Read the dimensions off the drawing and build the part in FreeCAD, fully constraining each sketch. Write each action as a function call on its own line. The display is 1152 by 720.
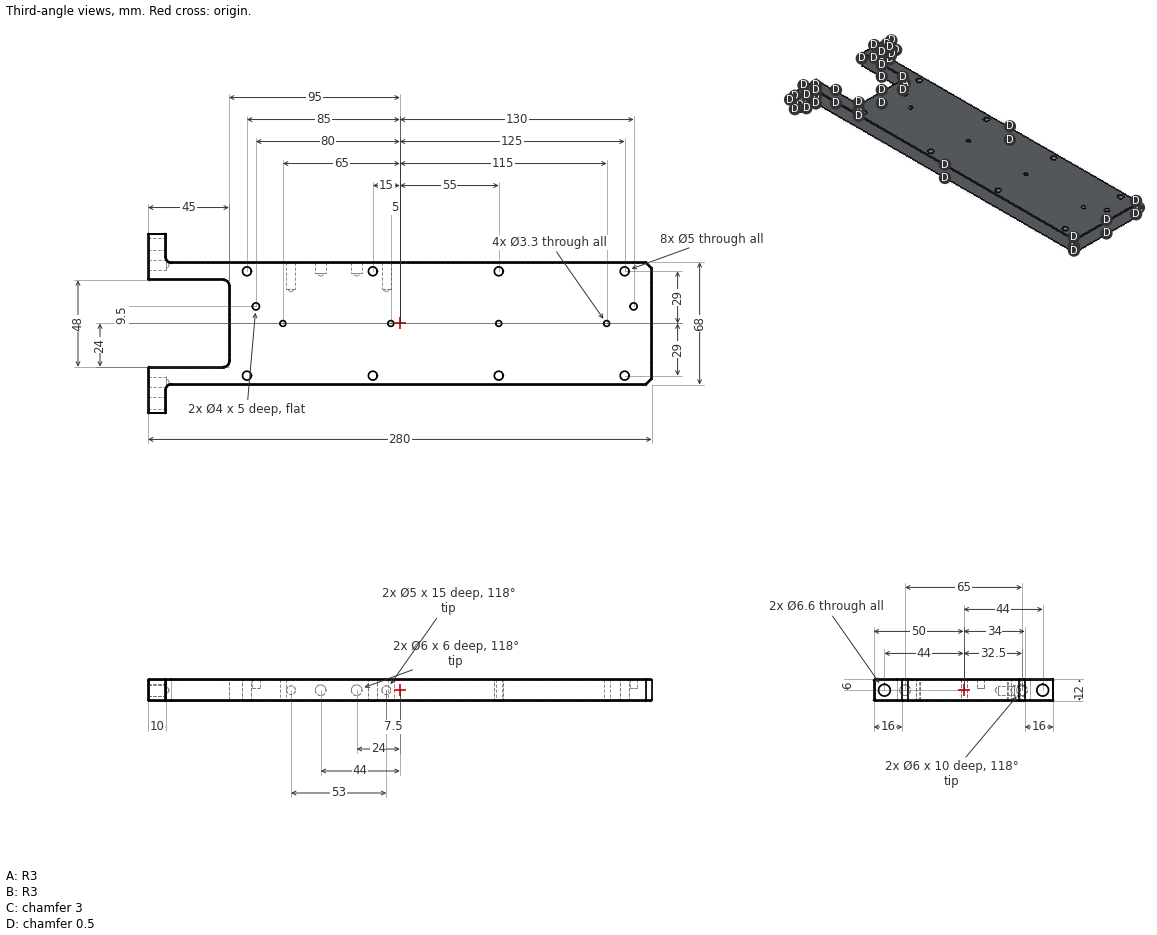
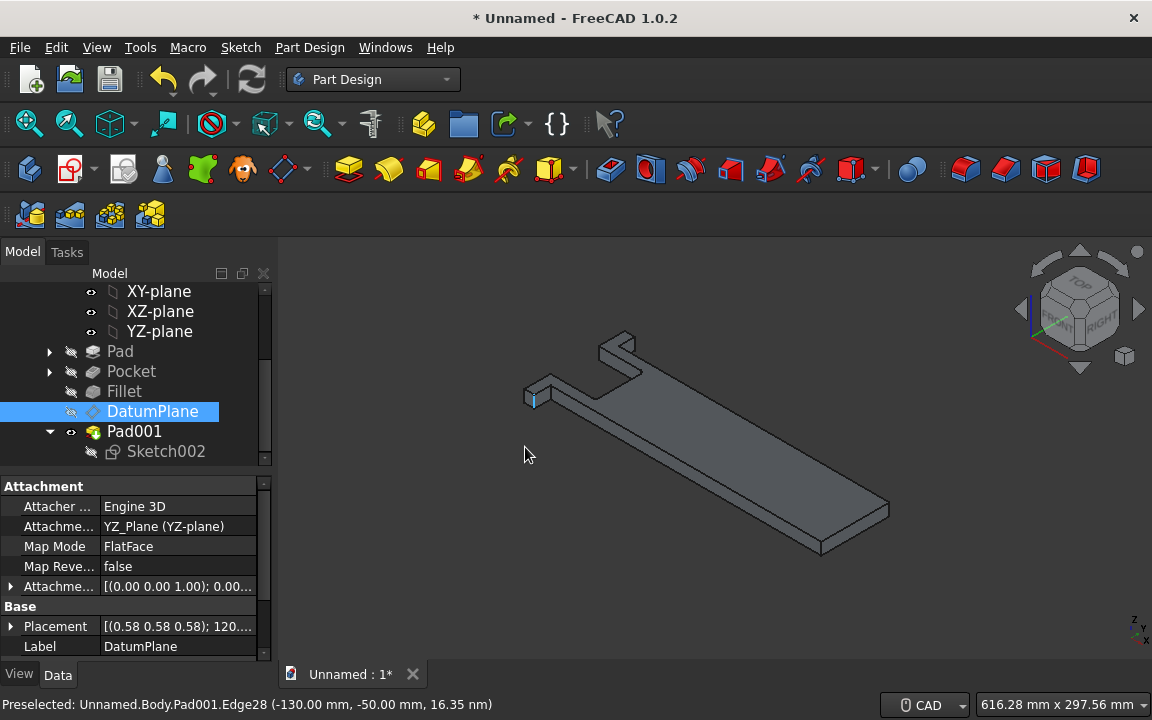
scroll(551, 391, up, 5)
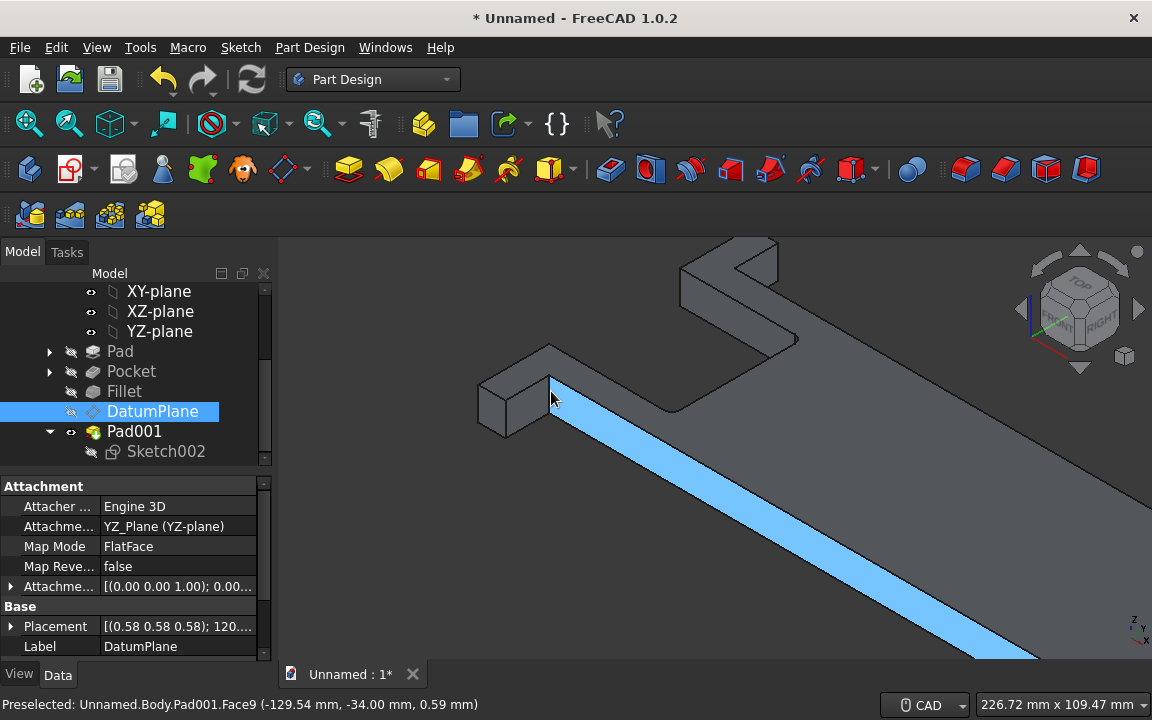
key(v)
key(f)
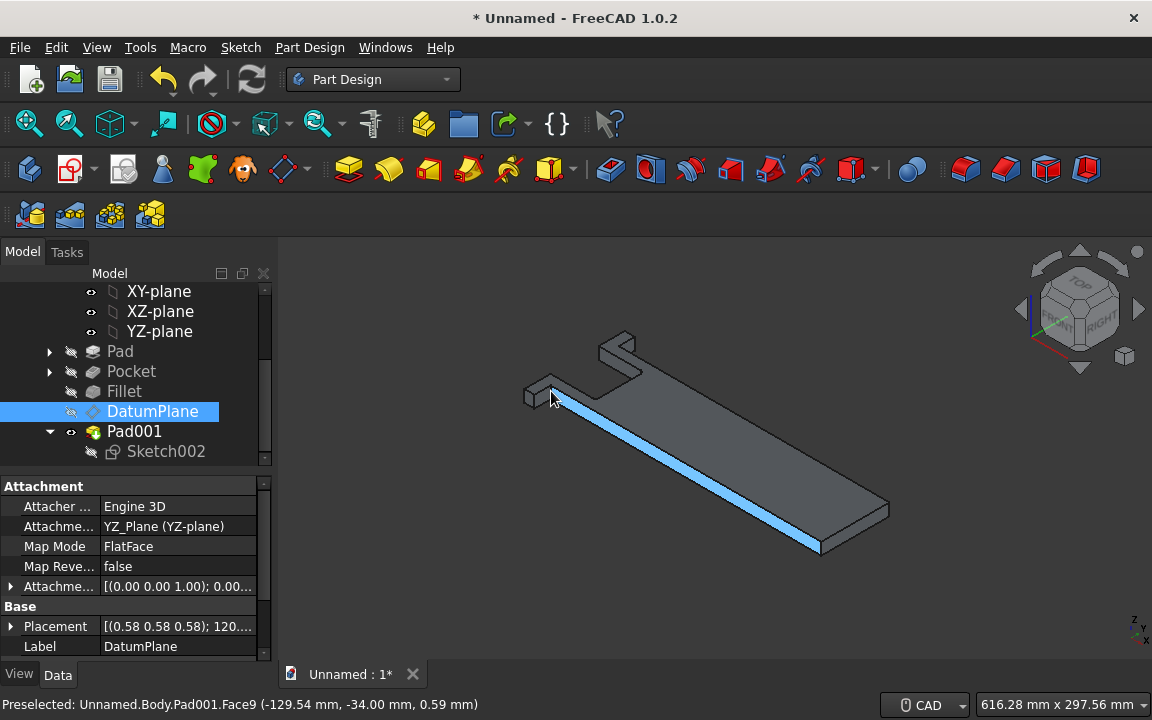
key(2)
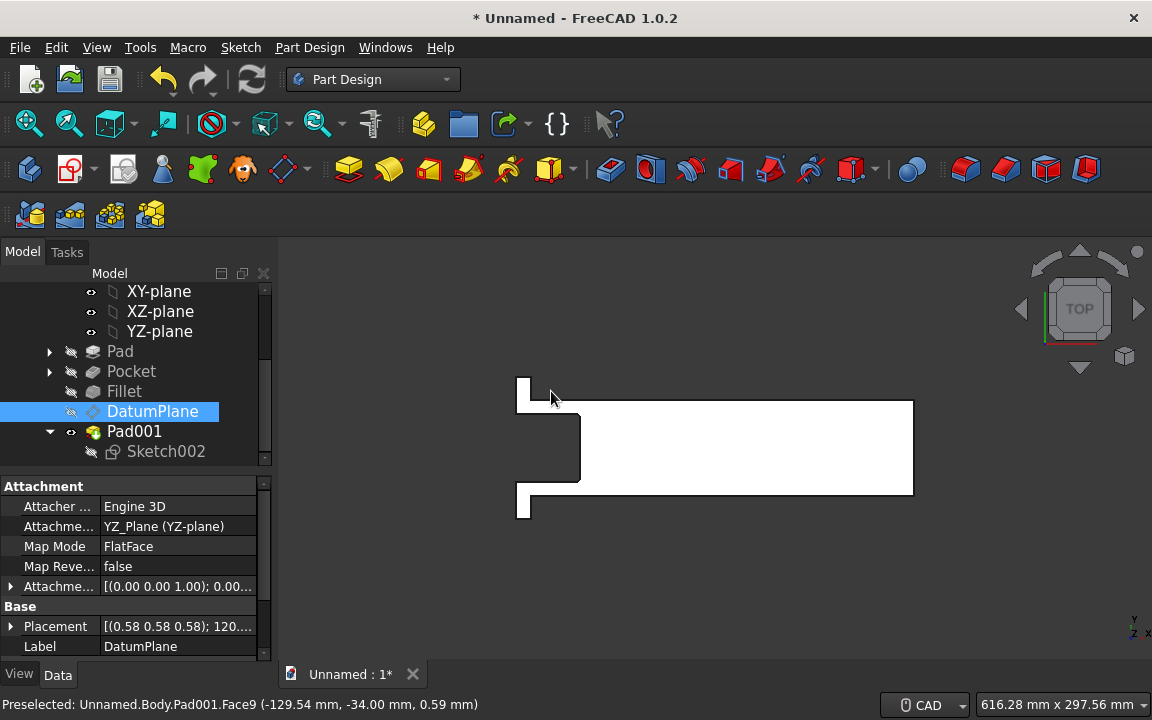
scroll(531, 495, up, 5)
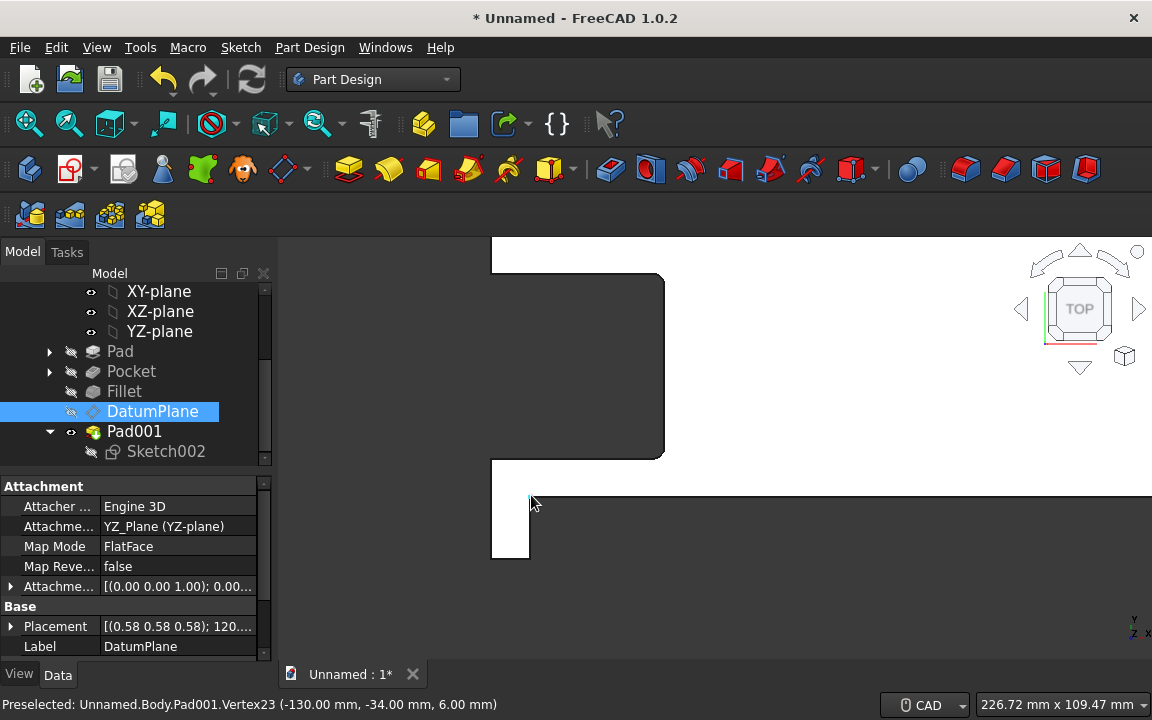
click(30, 124)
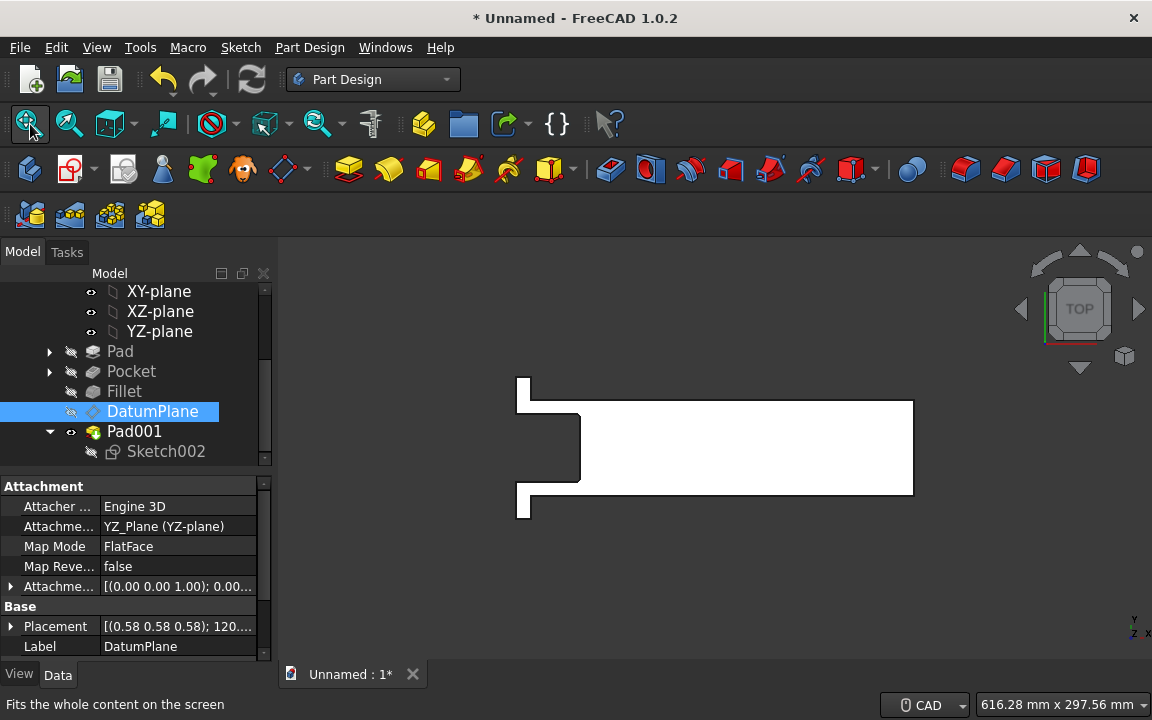
key(1)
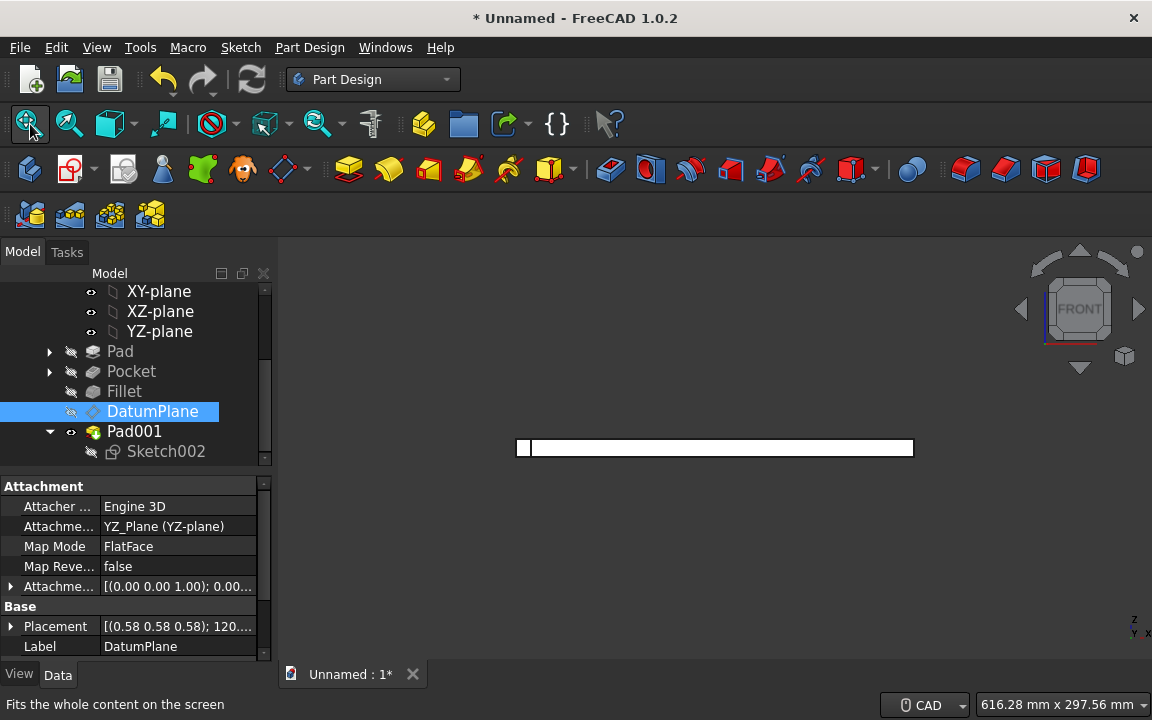
scroll(531, 447, up, 5)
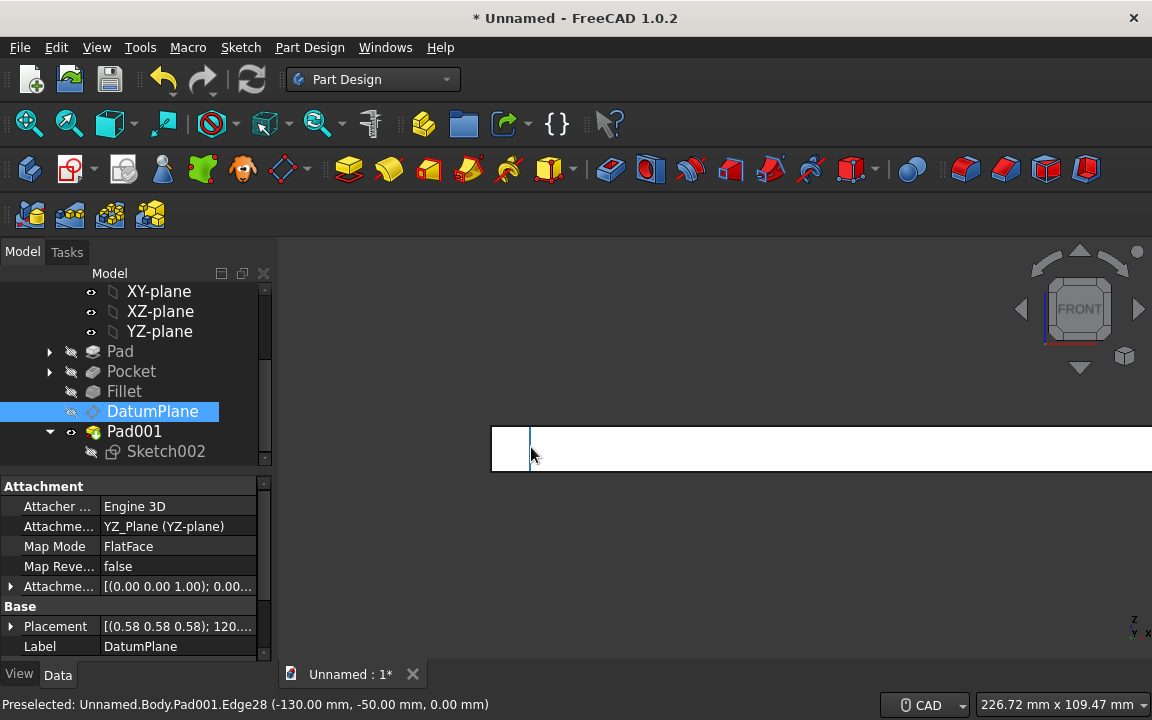
click(30, 124)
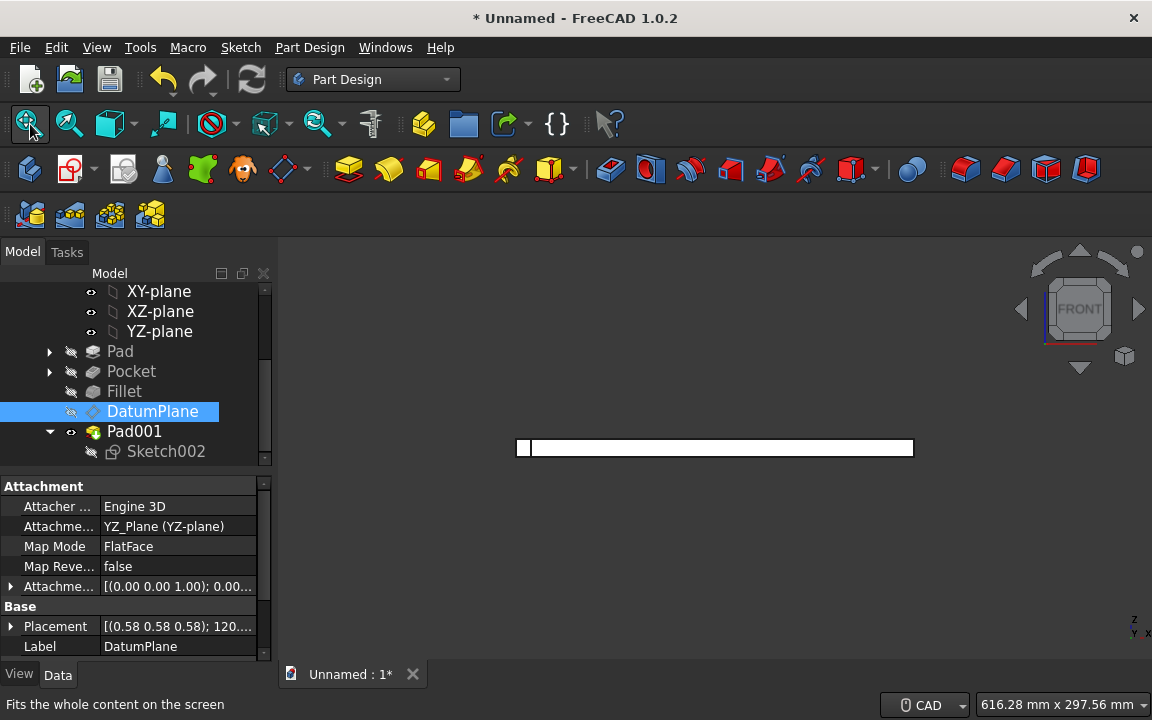
key(3)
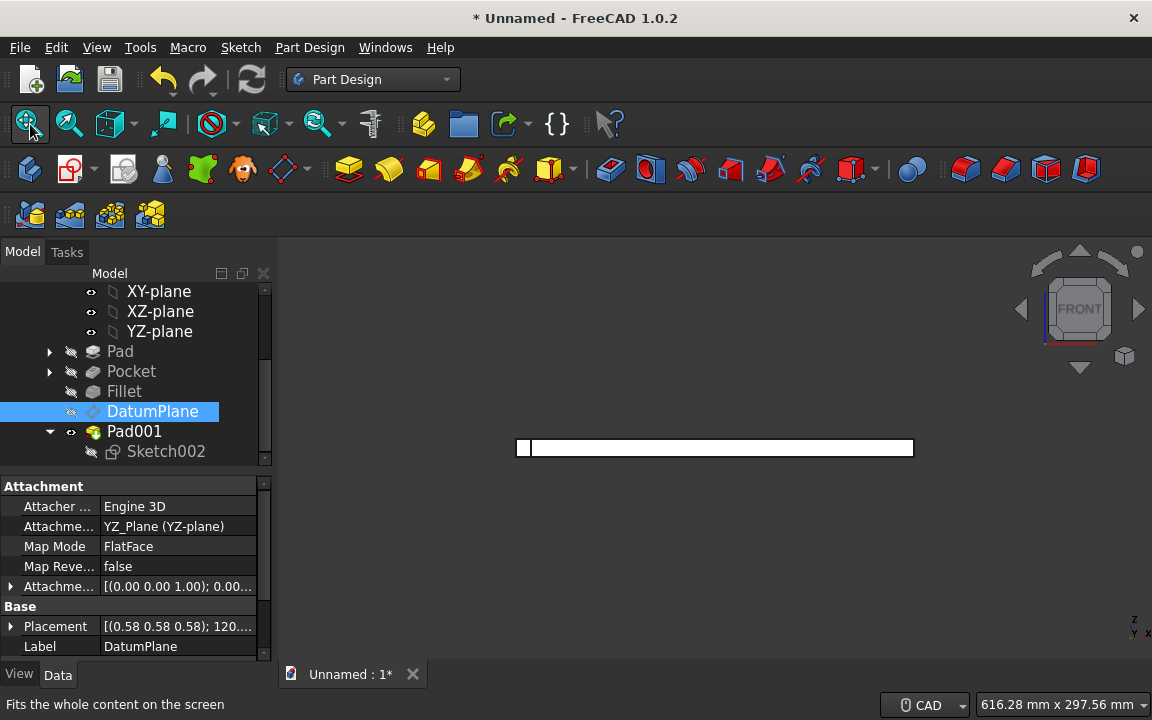
key(v)
key(f)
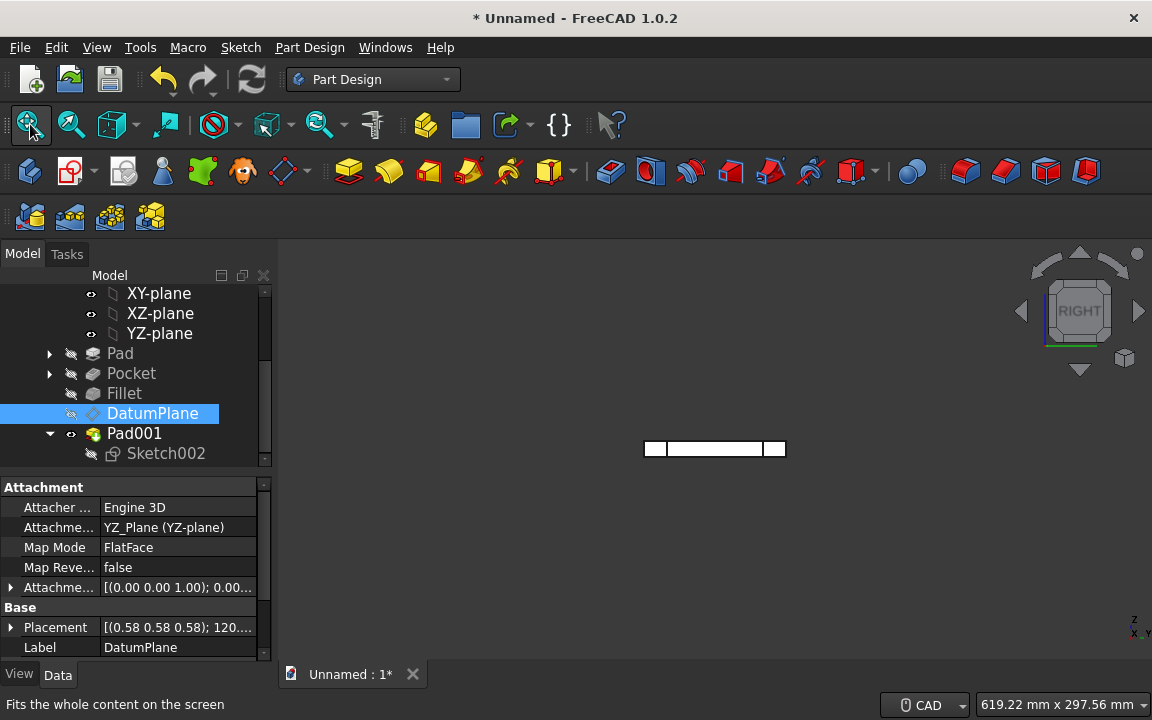
scroll(667, 448, up, 5)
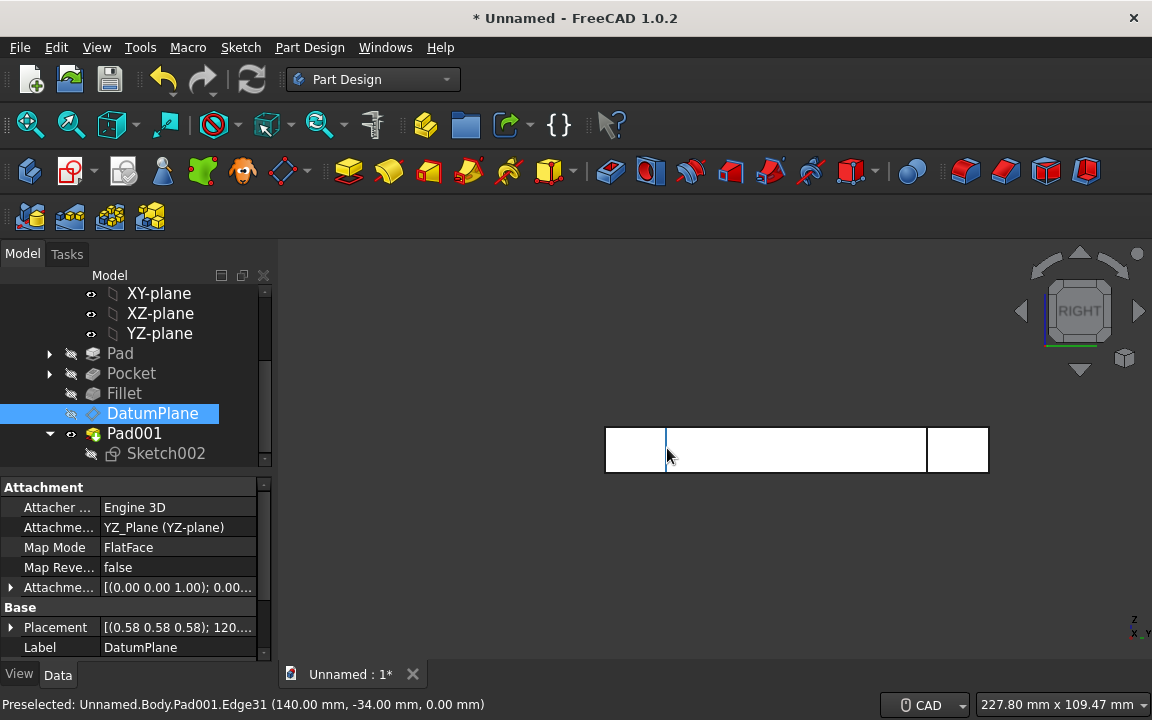
click(32, 126)